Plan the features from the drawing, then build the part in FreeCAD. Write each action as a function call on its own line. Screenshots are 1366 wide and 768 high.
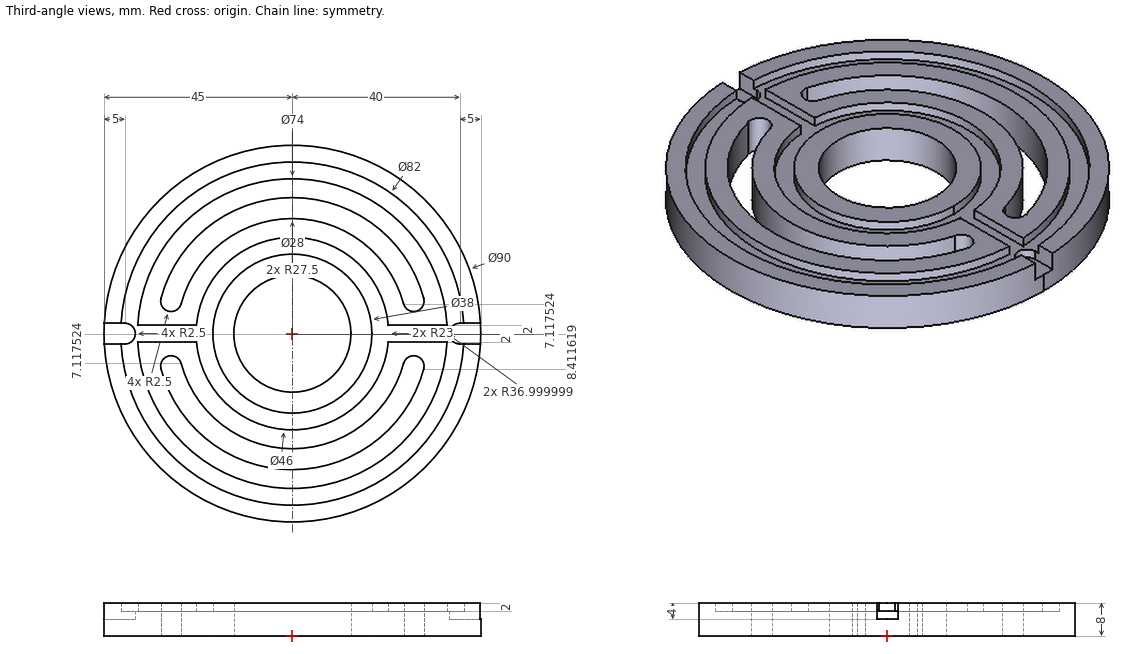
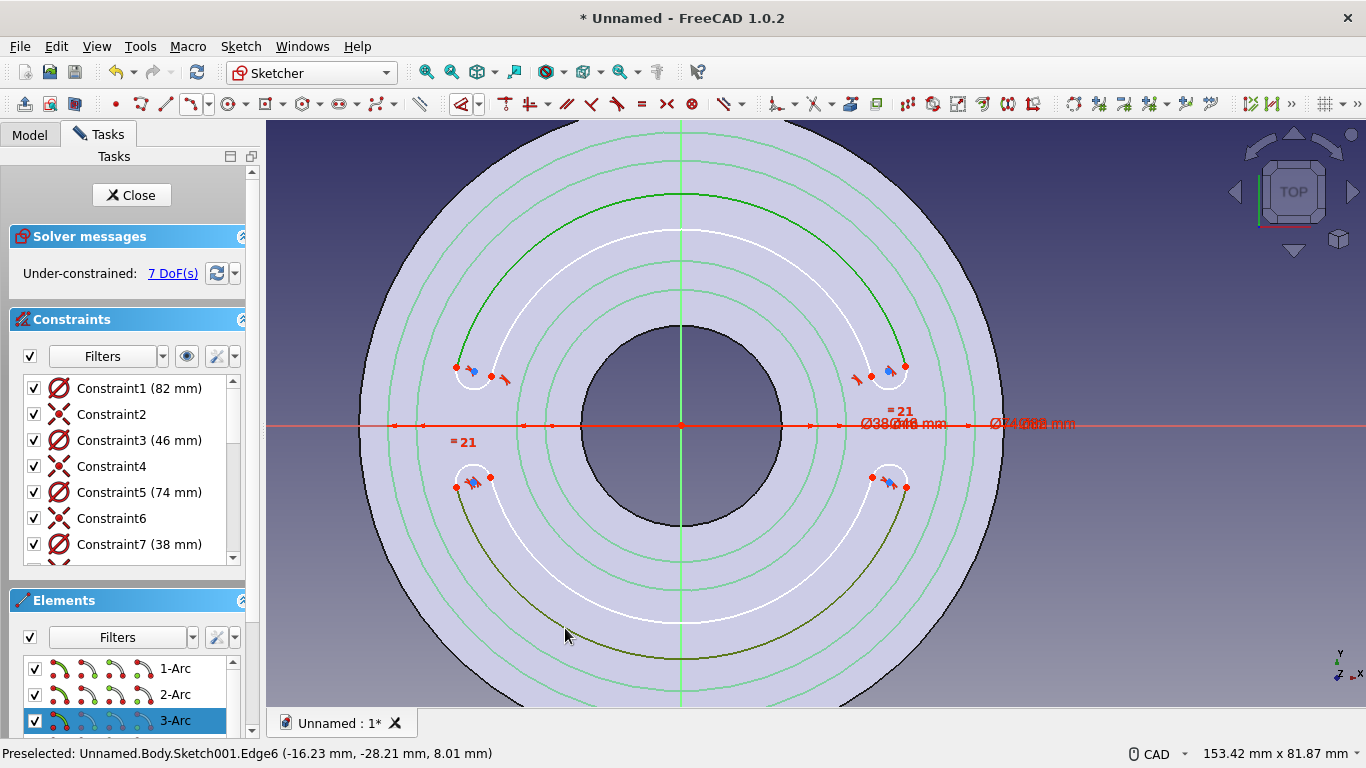
key(e)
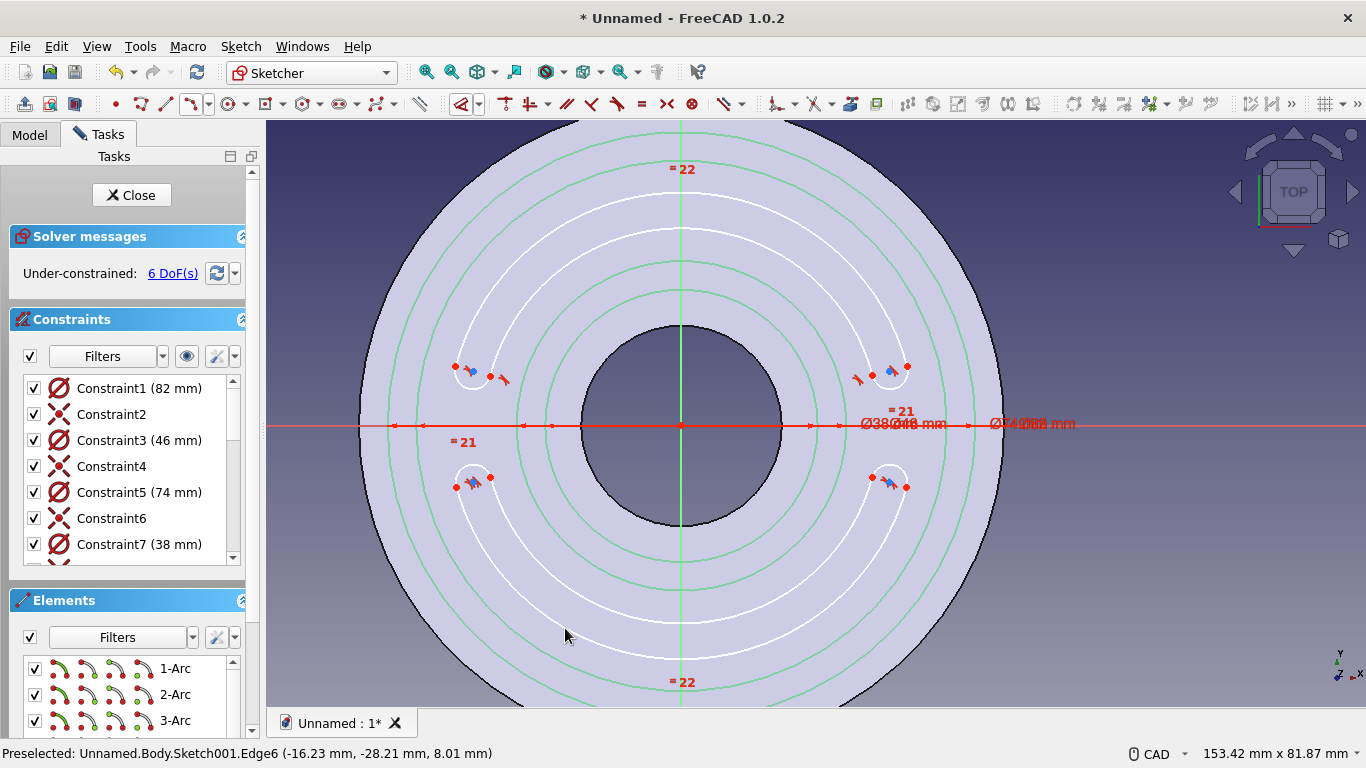
key(d)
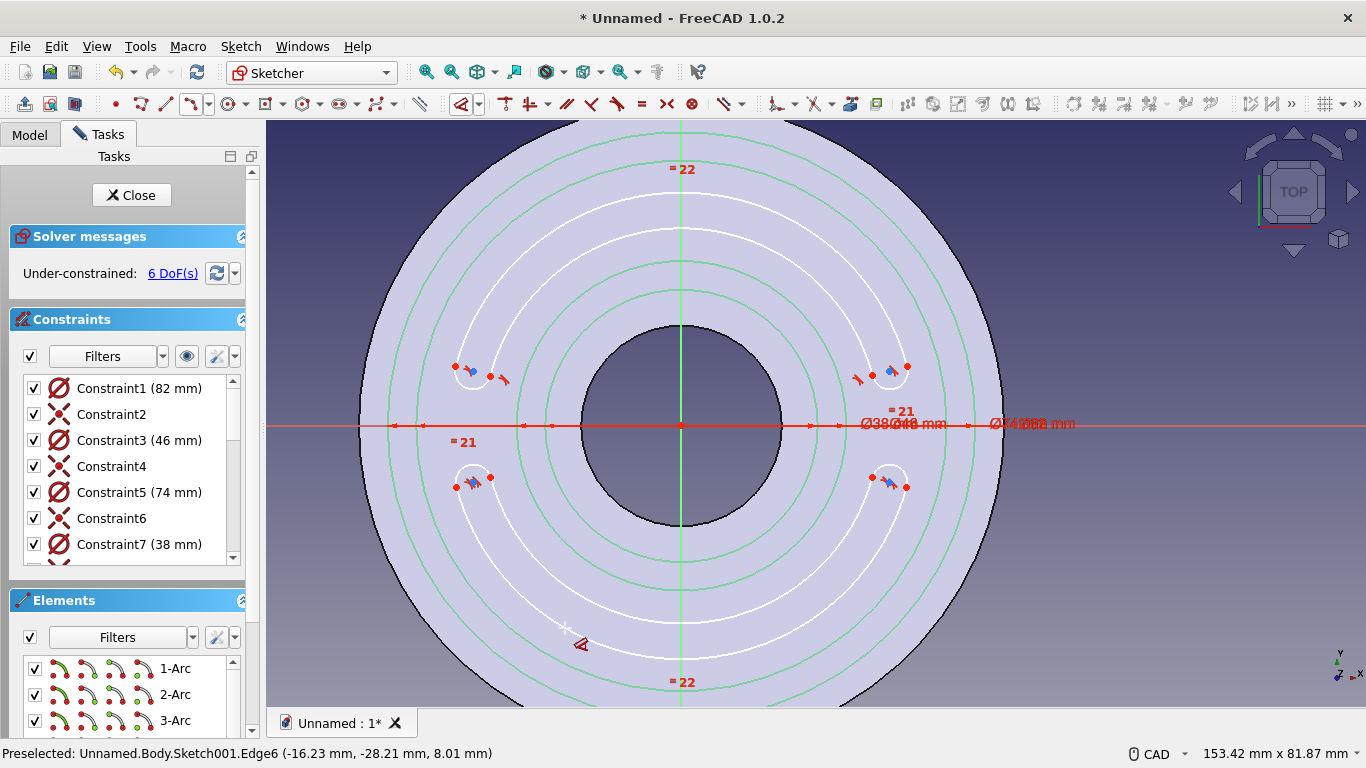
click(781, 255)
click(911, 416)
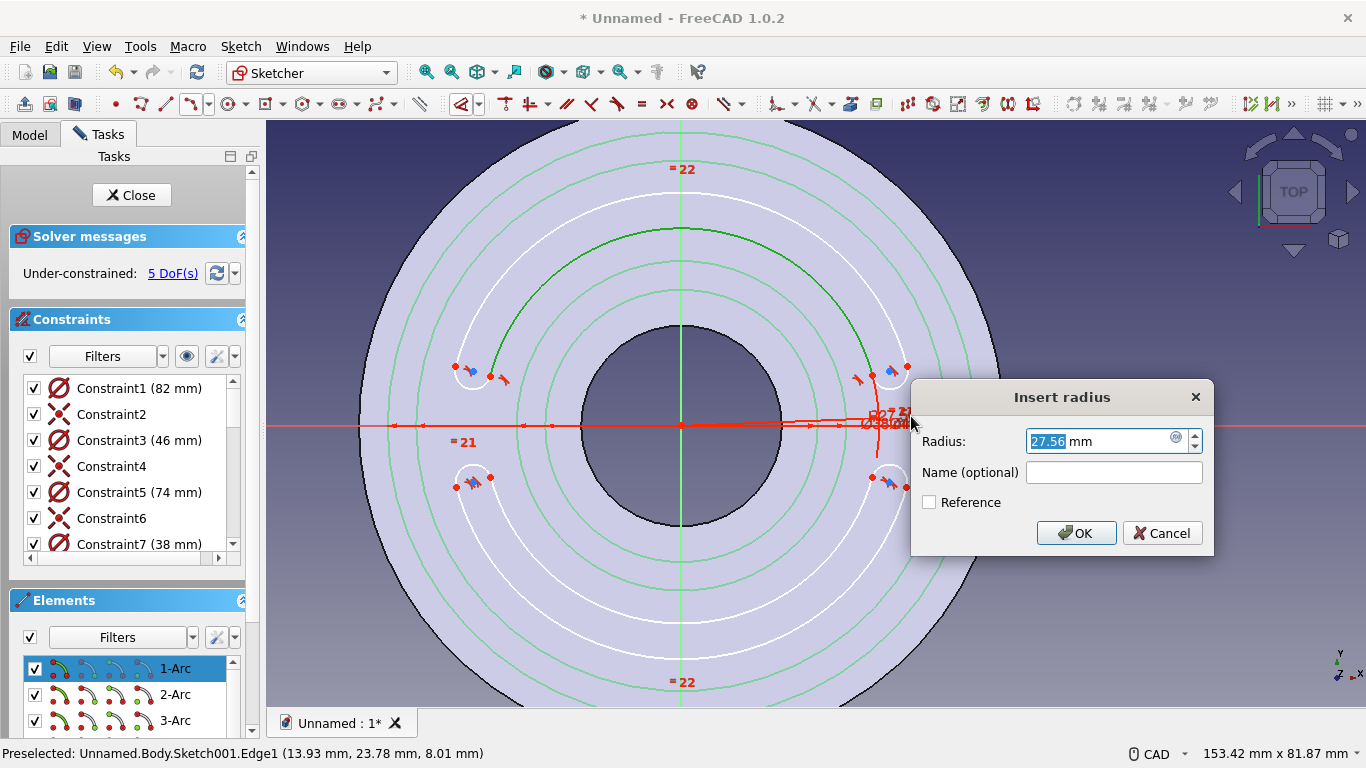
text(27.5)
key(Return)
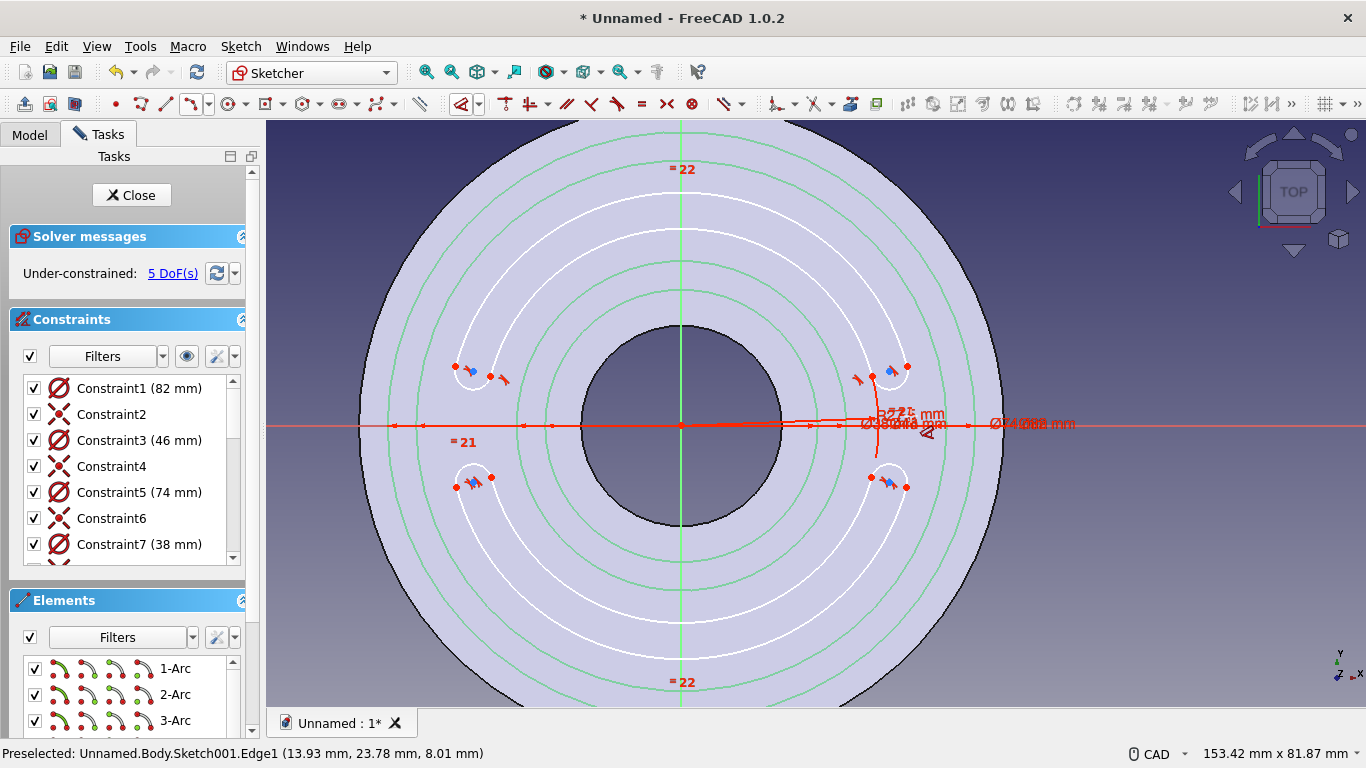
scroll(883, 388, up, 4)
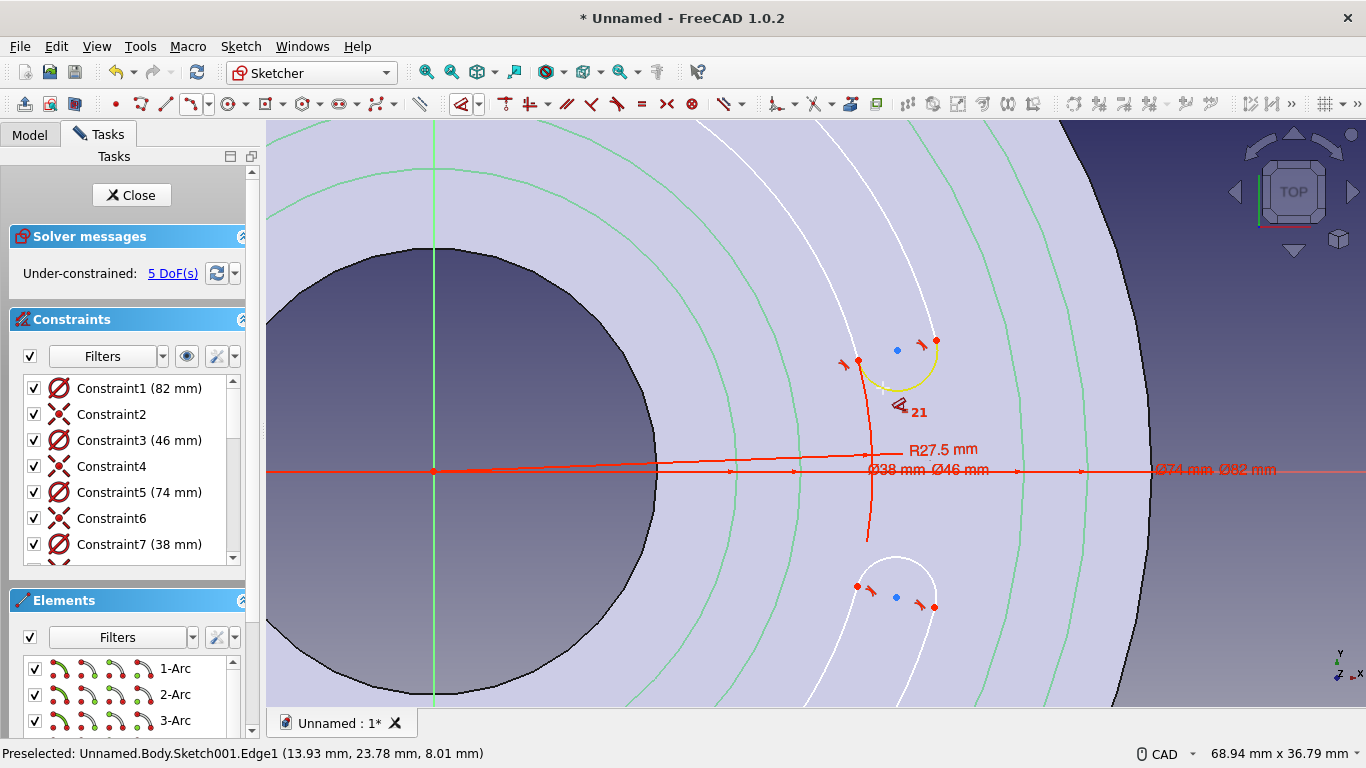
click(883, 388)
click(872, 418)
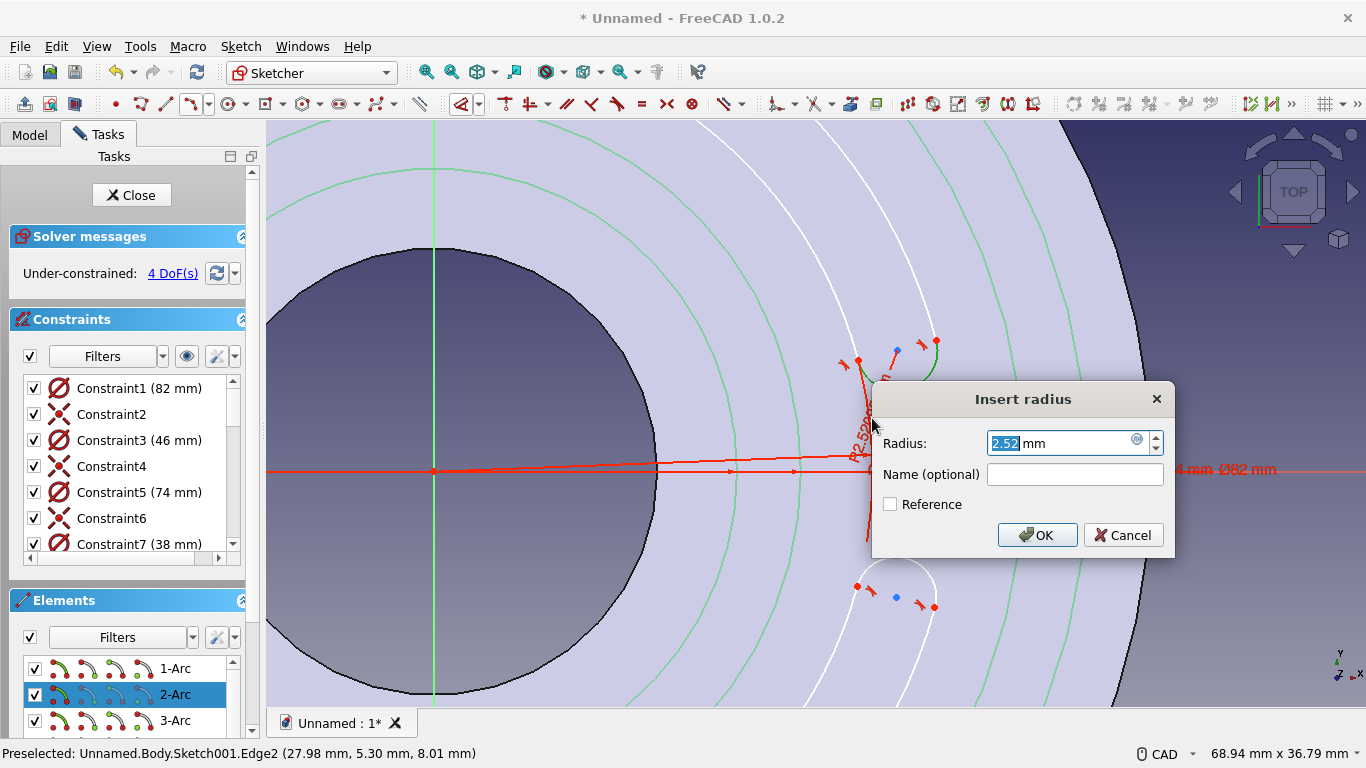
text(2.5)
key(Return)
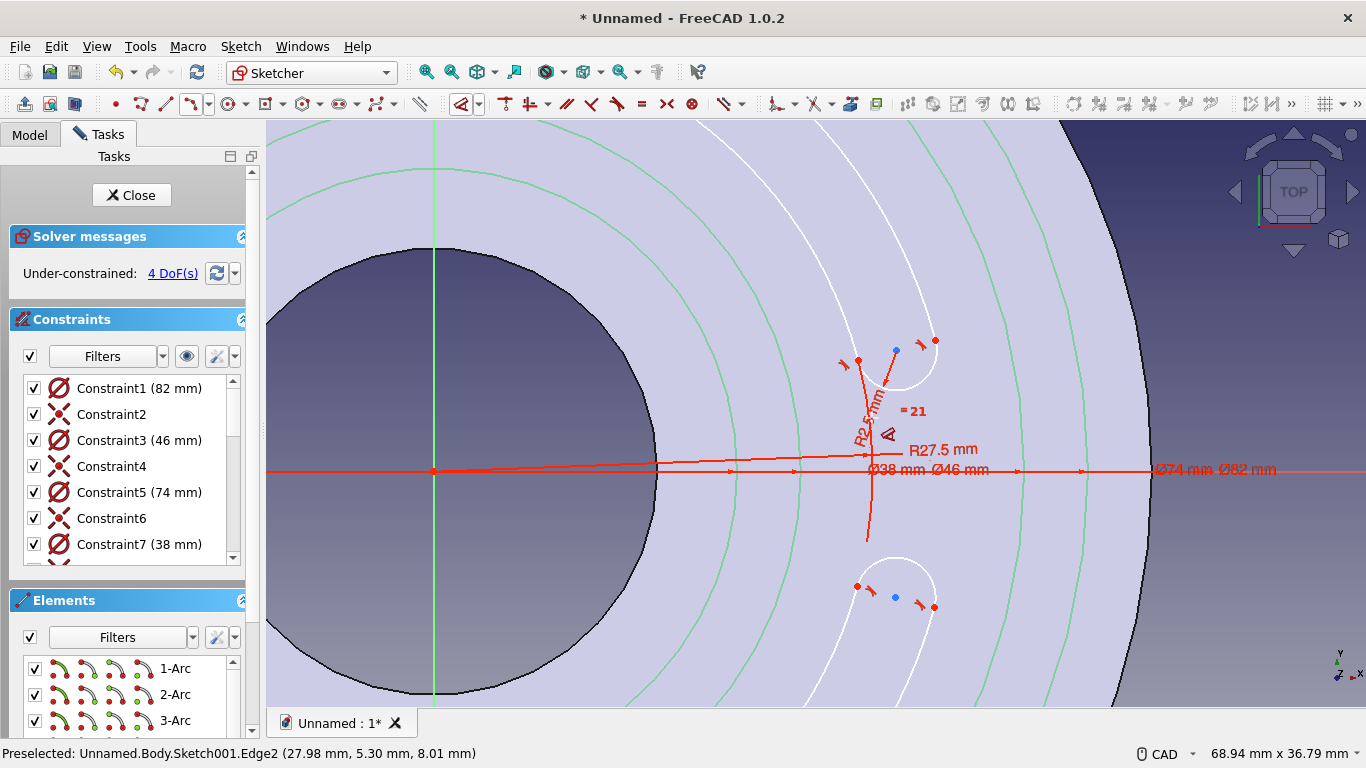
click(858, 361)
click(400, 416)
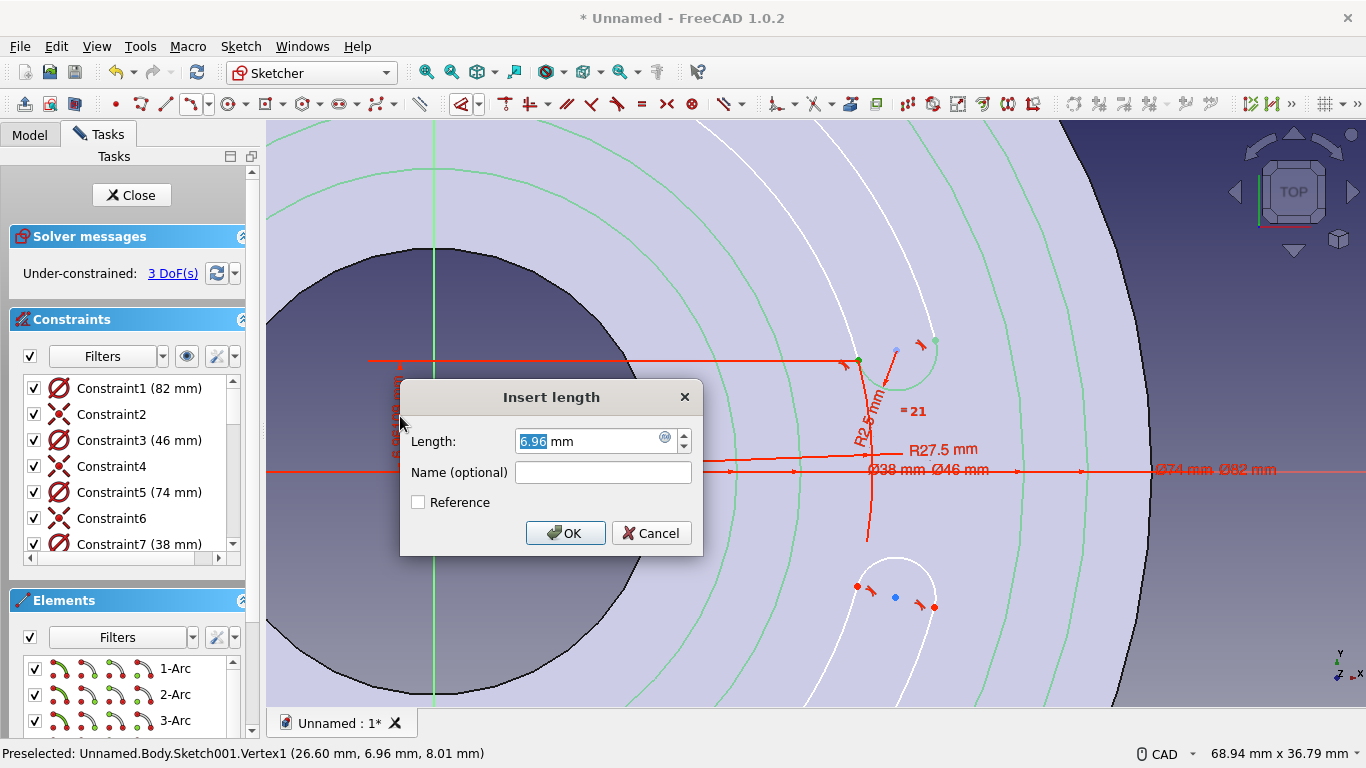
text(7.117524)
key(Return)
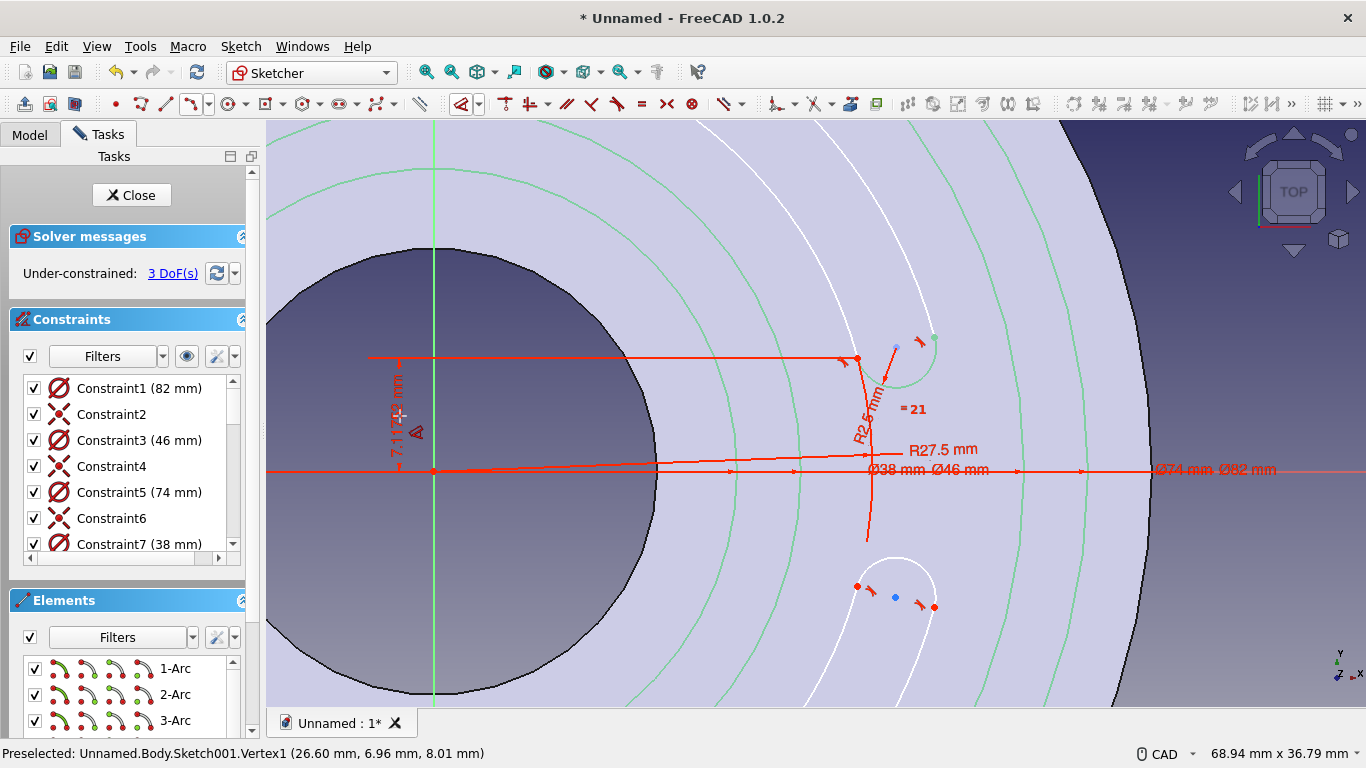
scroll(883, 388, down, 6)